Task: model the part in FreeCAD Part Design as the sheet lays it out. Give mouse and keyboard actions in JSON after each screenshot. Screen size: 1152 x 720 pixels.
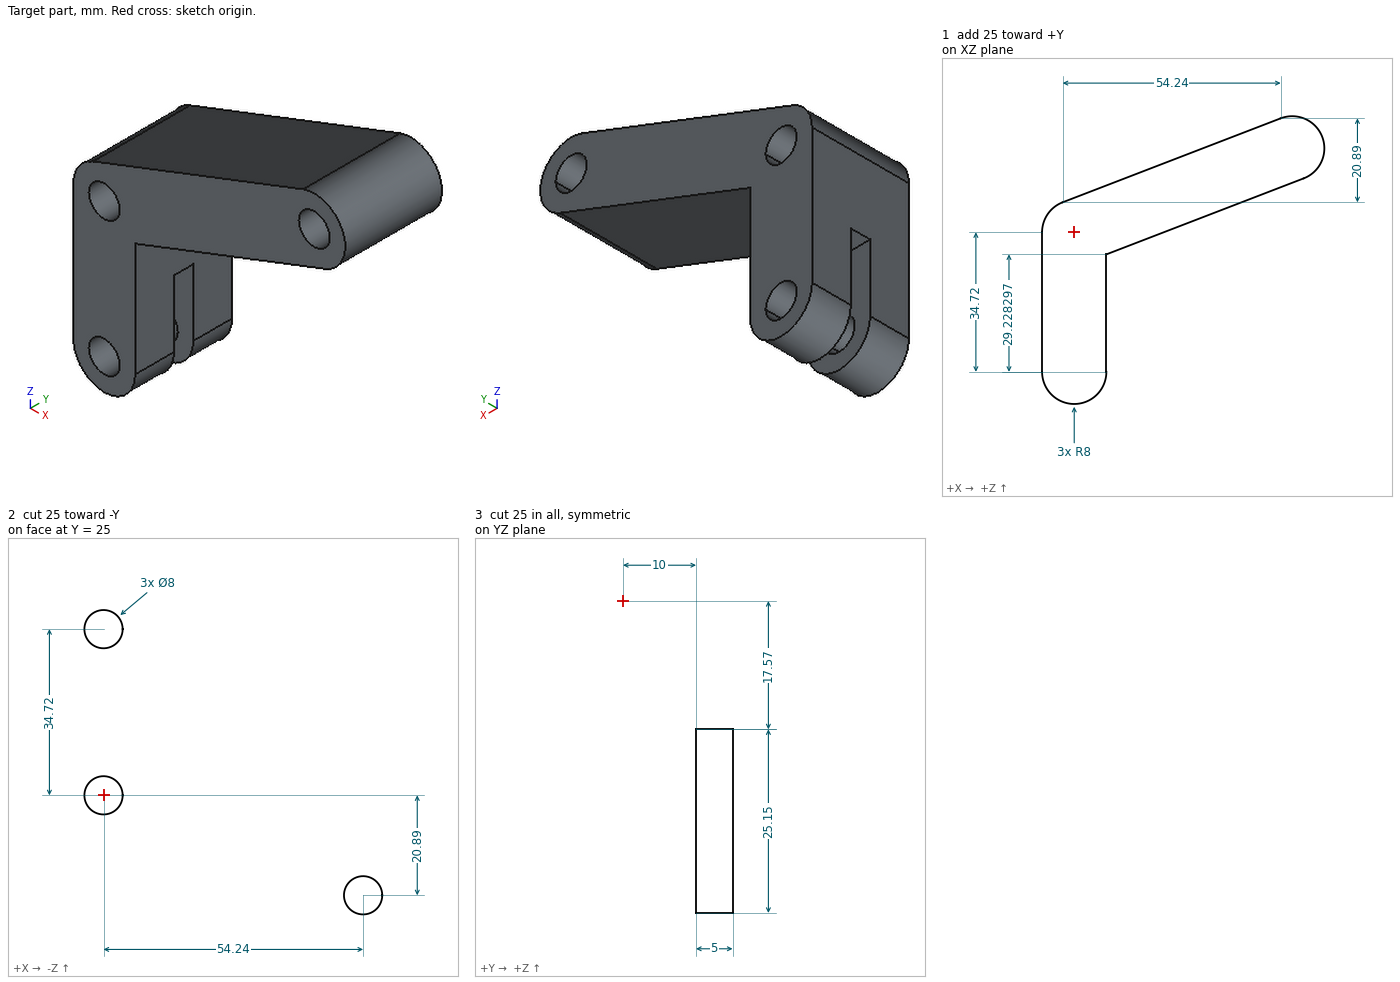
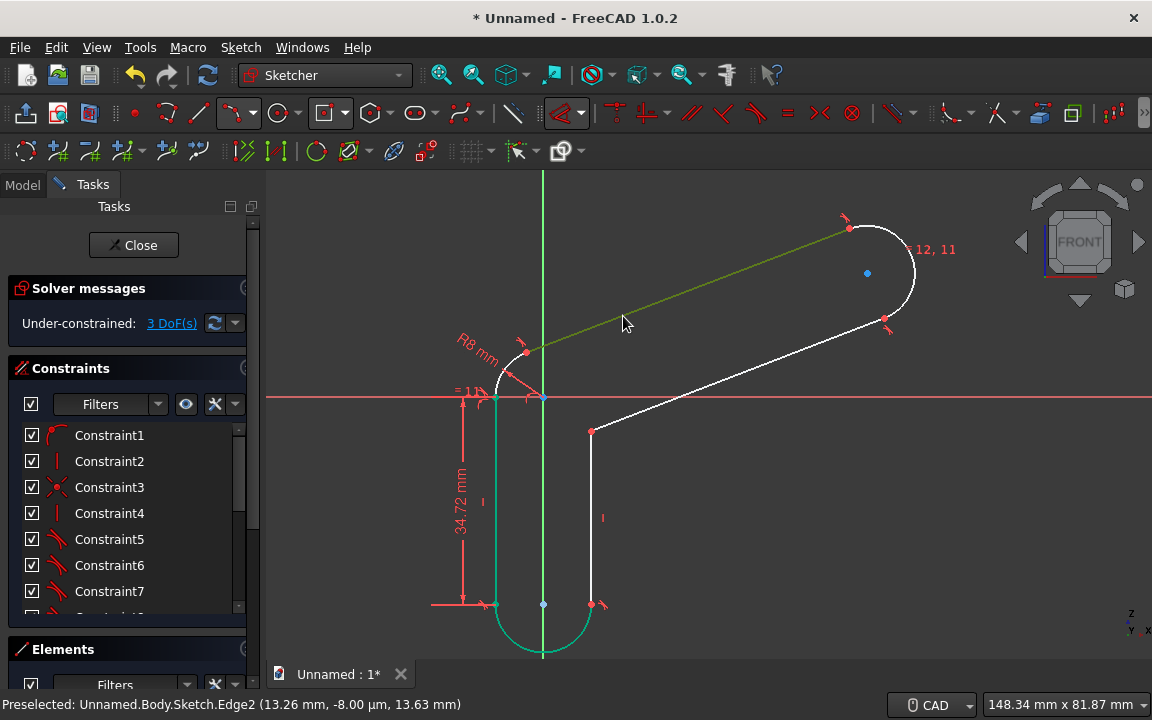
{"action": "left_click", "coordinate": [584, 114]}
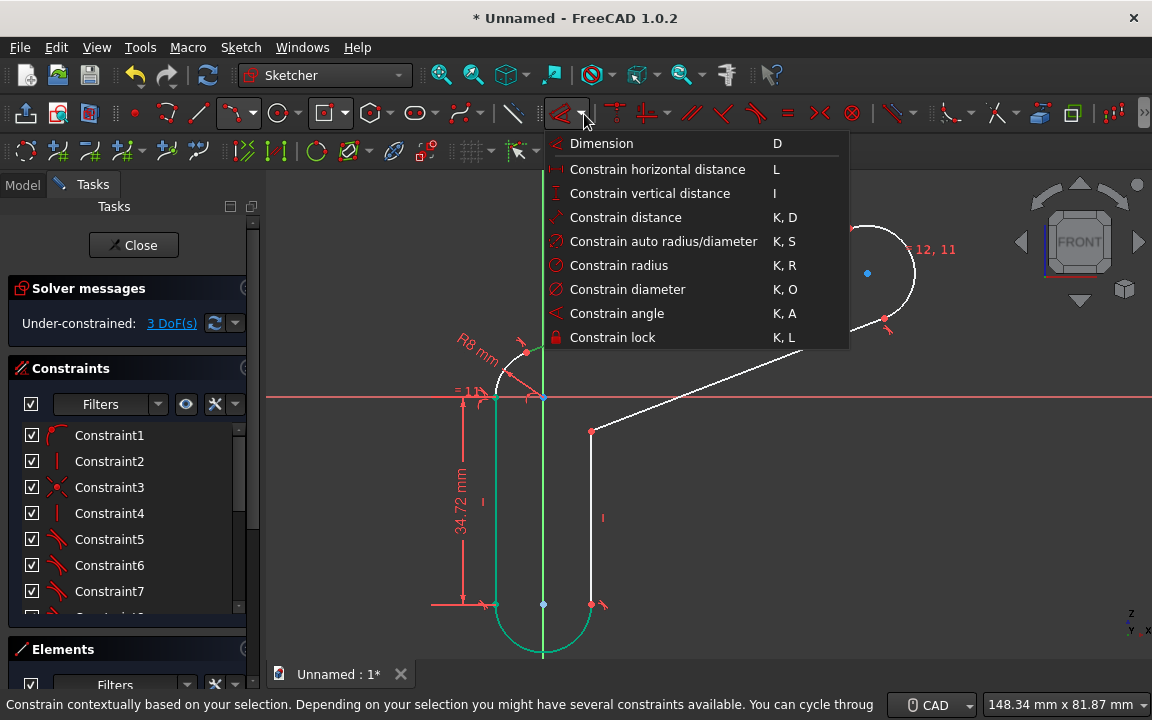
{"action": "left_click", "coordinate": [697, 169]}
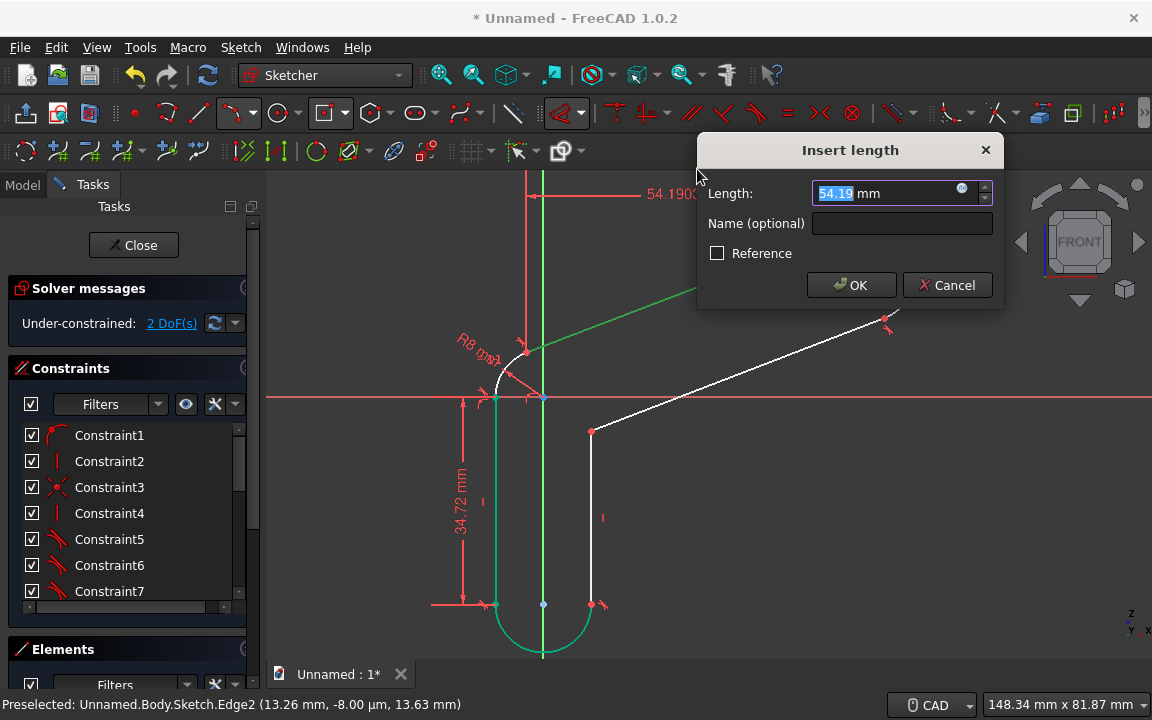
{"action": "type", "text": "54.24"}
{"action": "key", "text": "Return"}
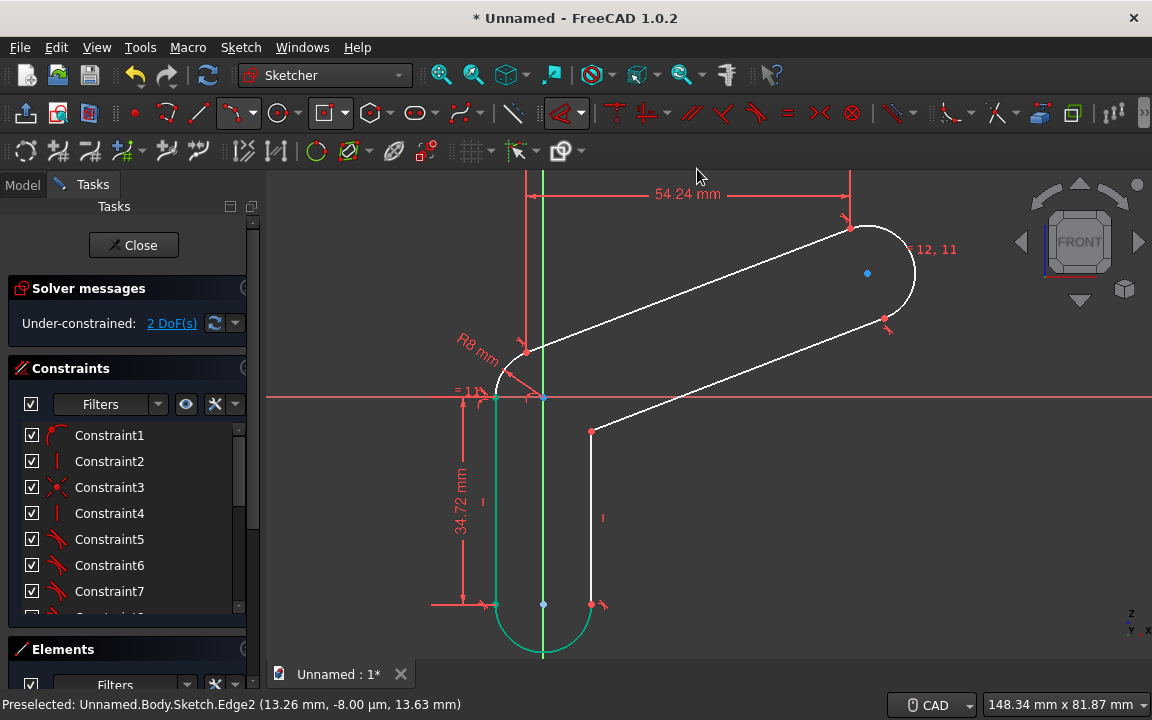
{"action": "left_click", "coordinate": [624, 316]}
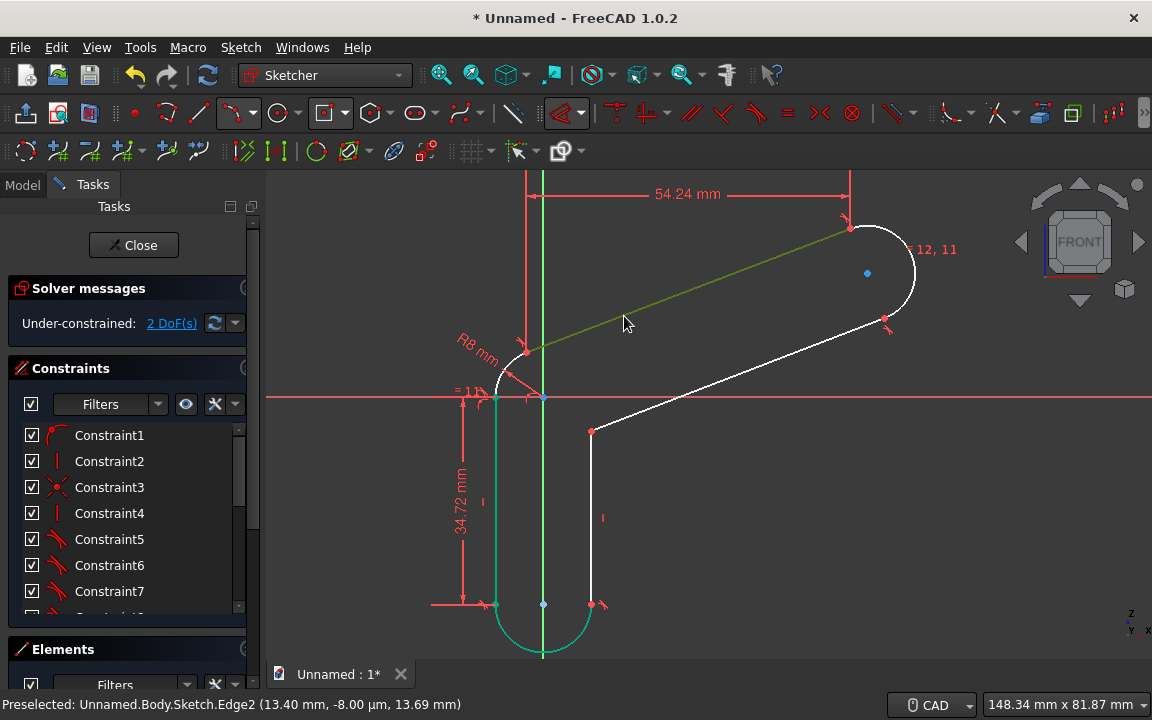
{"action": "left_click", "coordinate": [584, 114]}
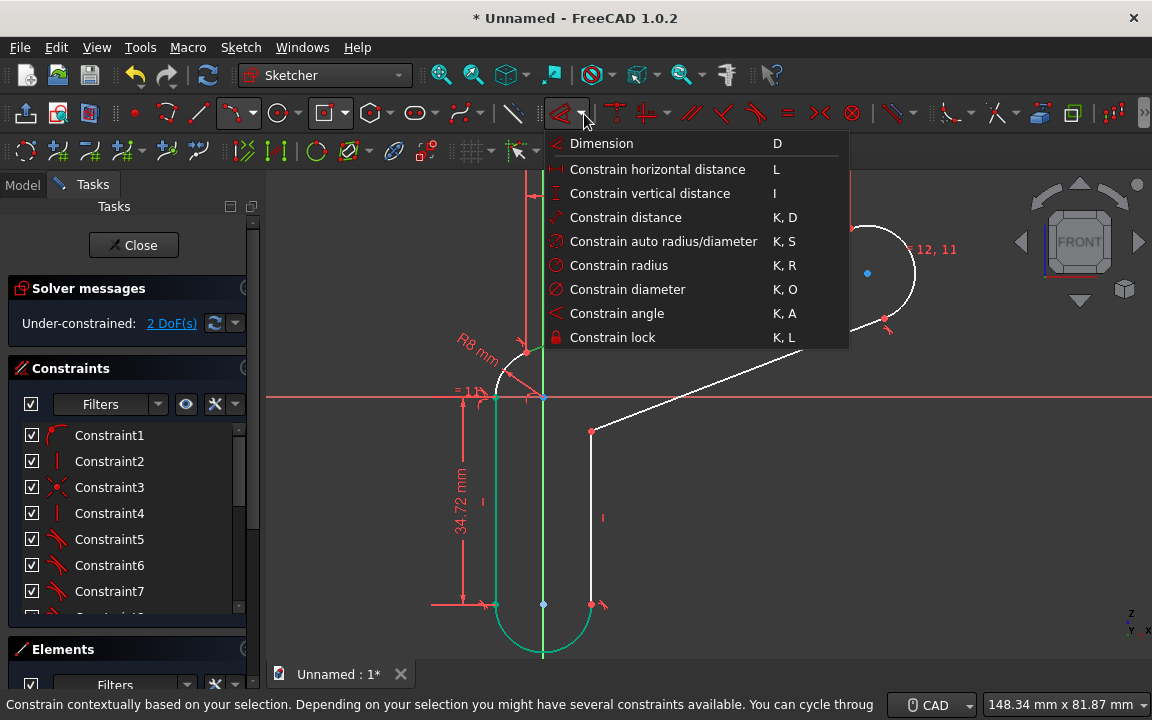
{"action": "left_click", "coordinate": [697, 193]}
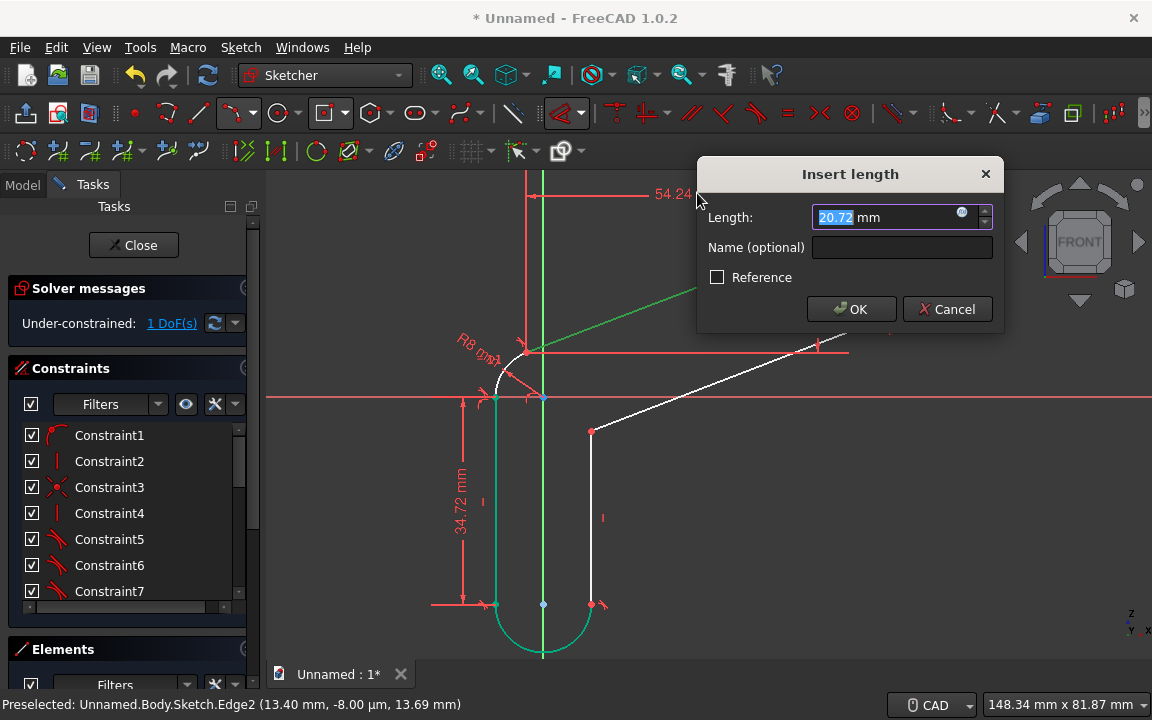
{"action": "type", "text": "20.89"}
{"action": "key", "text": "Return"}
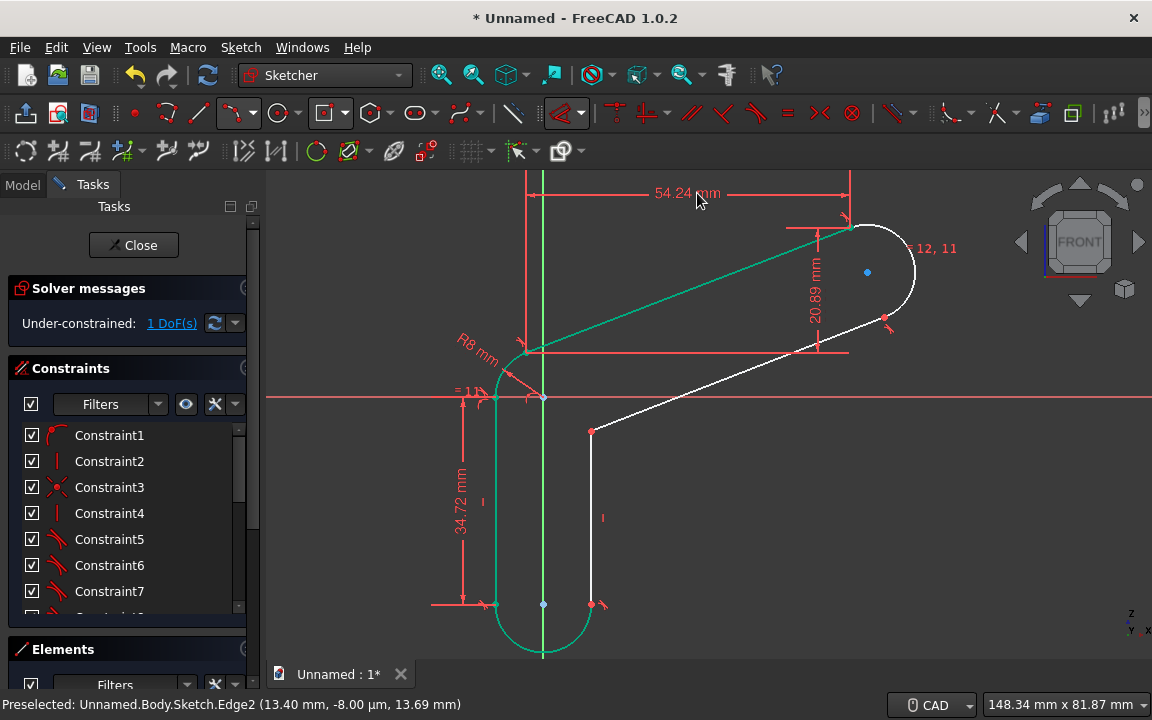
{"action": "left_click", "coordinate": [591, 483]}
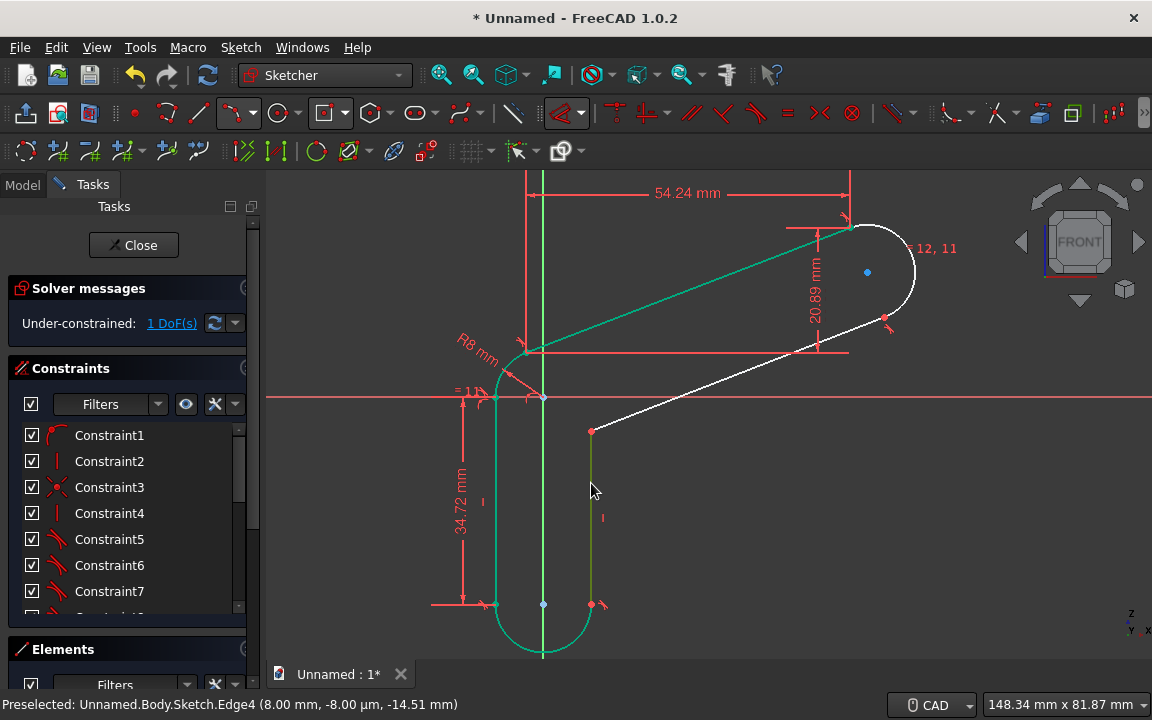
{"action": "left_click", "coordinate": [584, 114]}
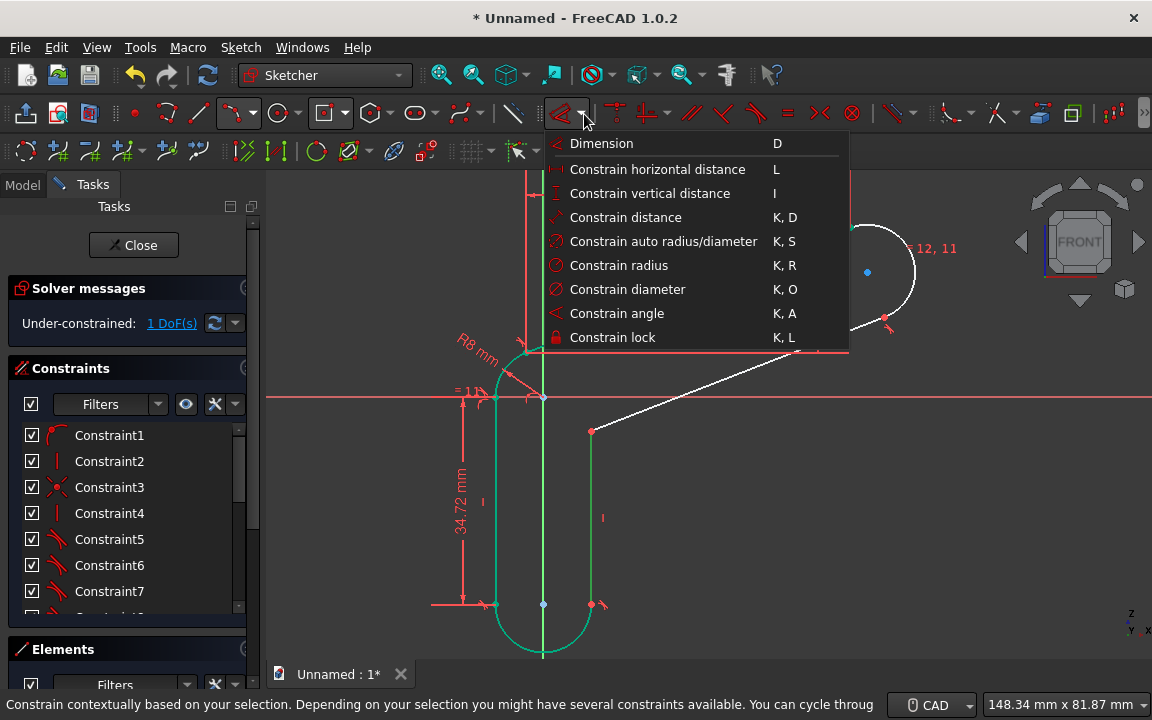
{"action": "left_click", "coordinate": [697, 193]}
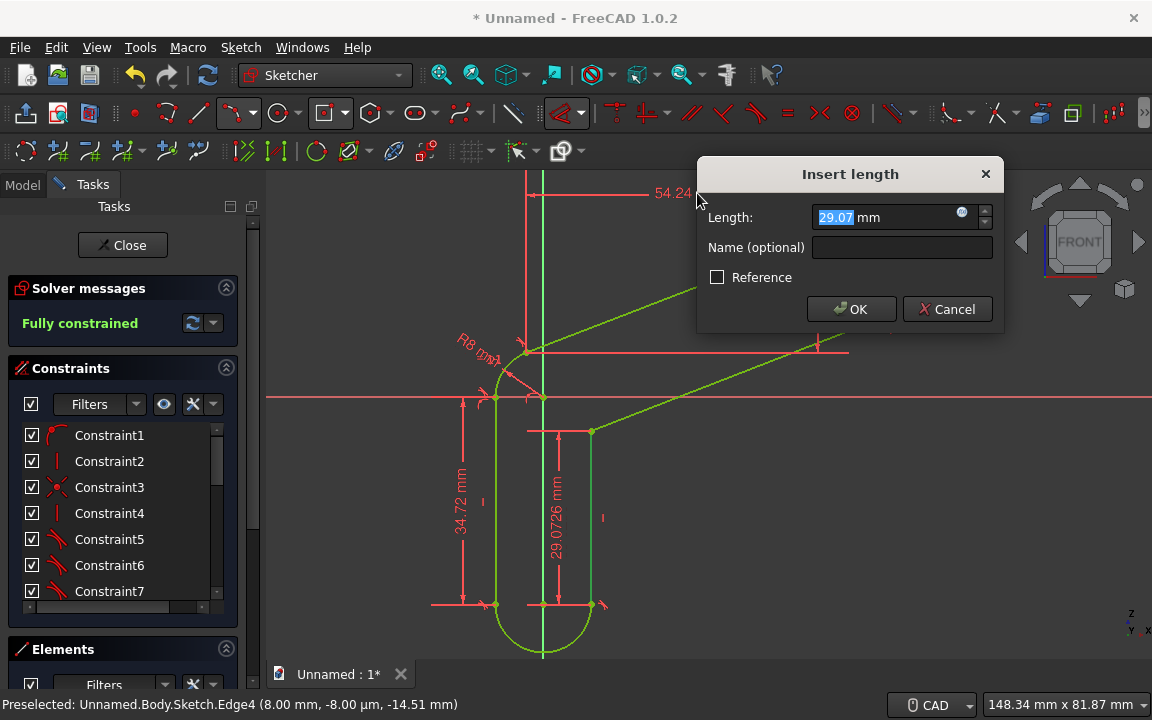
{"action": "type", "text": "29.228297"}
{"action": "key", "text": "Return"}